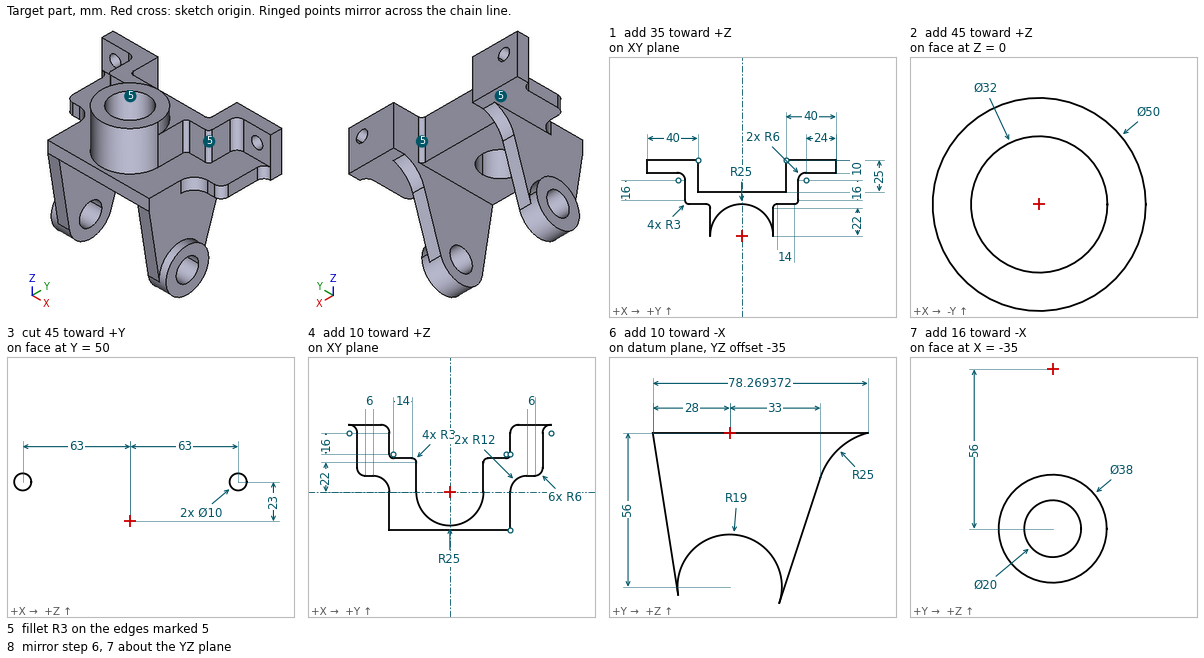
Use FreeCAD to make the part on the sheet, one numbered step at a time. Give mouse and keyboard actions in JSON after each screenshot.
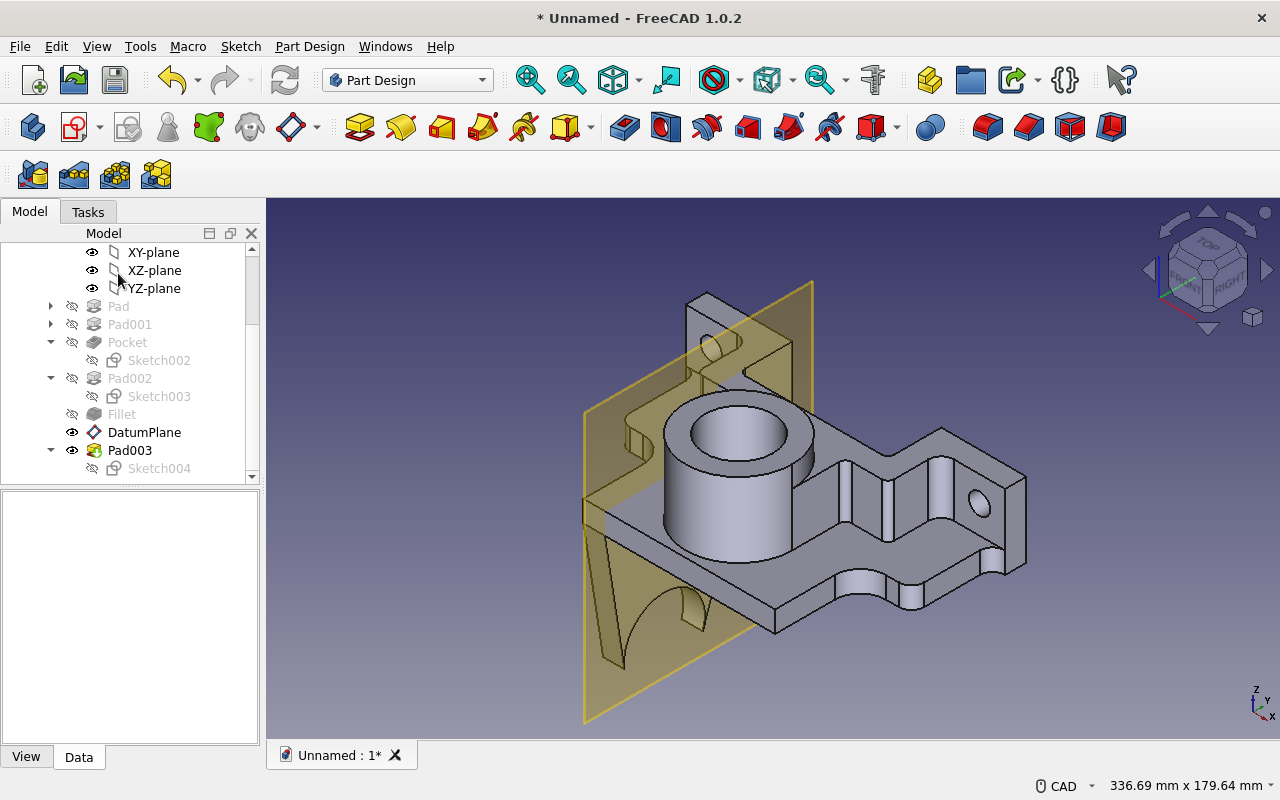
{"action": "left_click", "coordinate": [117, 432]}
{"action": "key", "text": "space"}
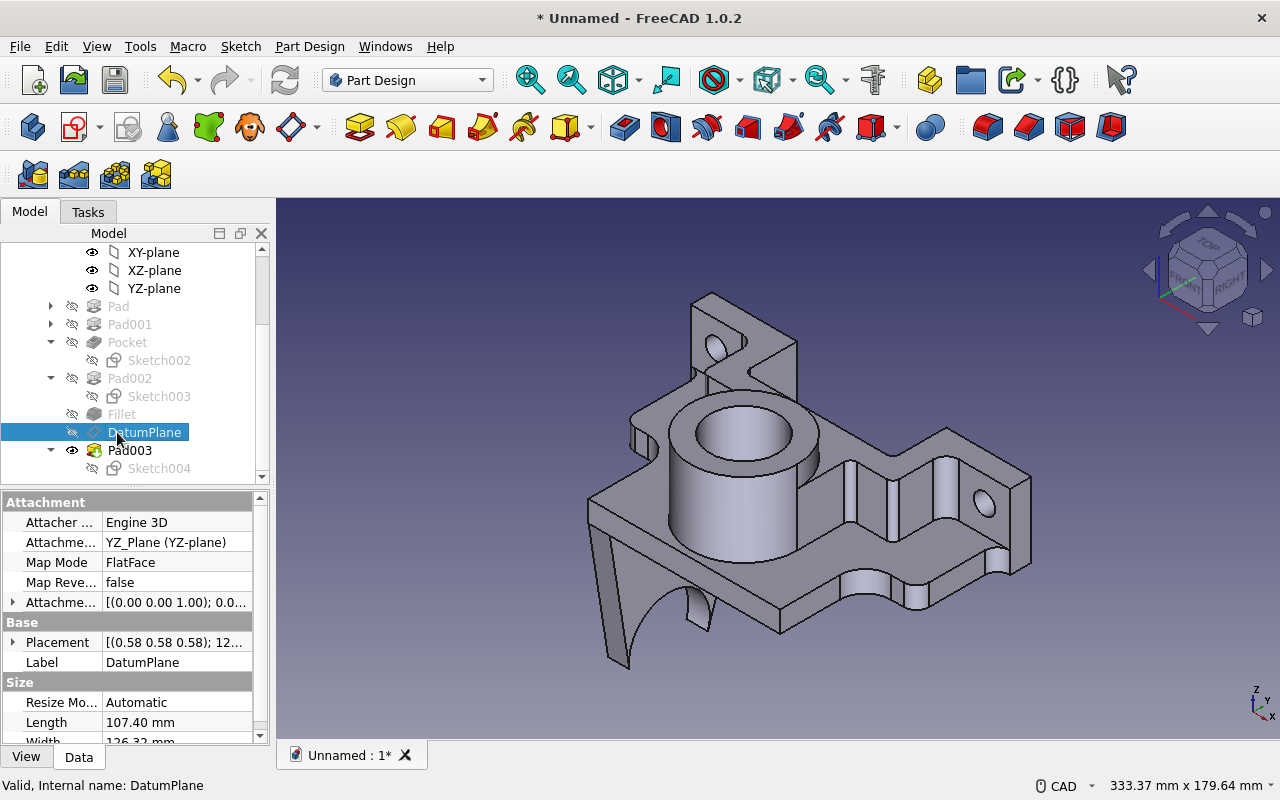
{"action": "left_click", "coordinate": [531, 80]}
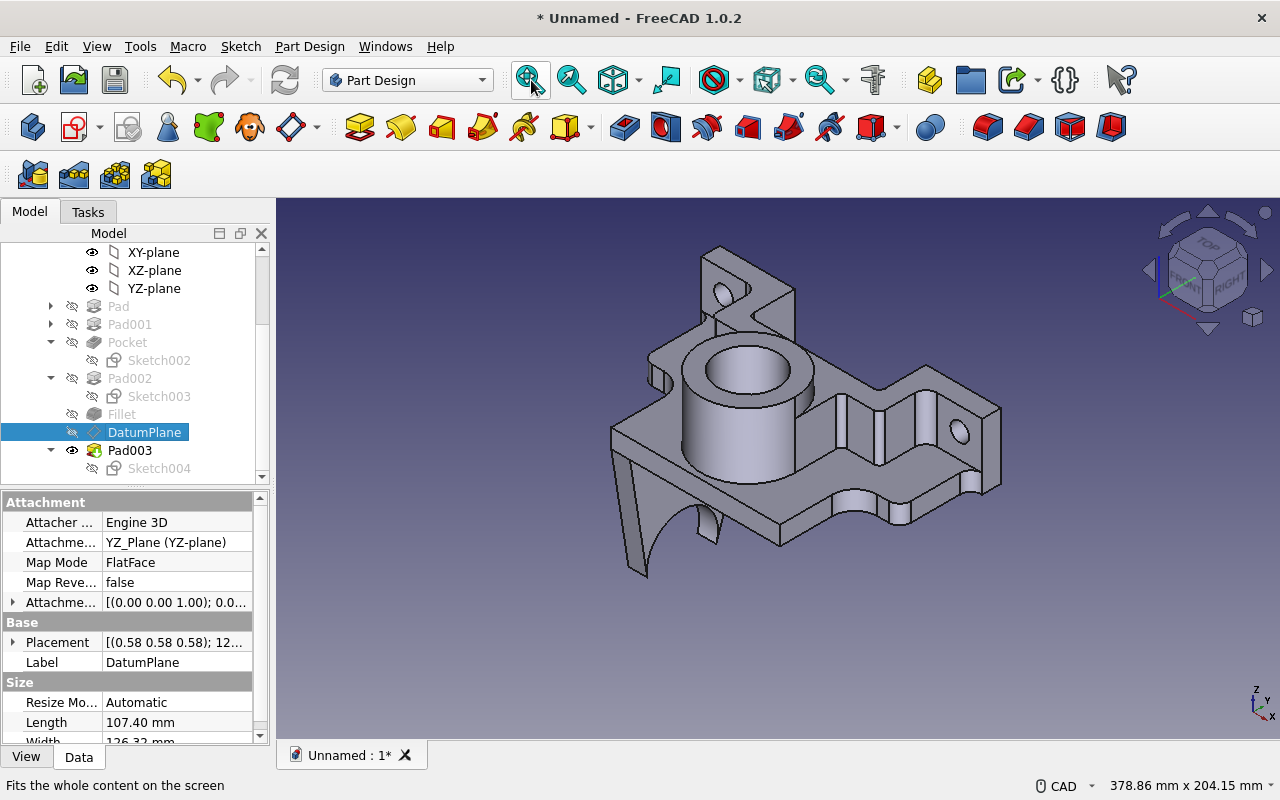
{"action": "left_click", "coordinate": [665, 498]}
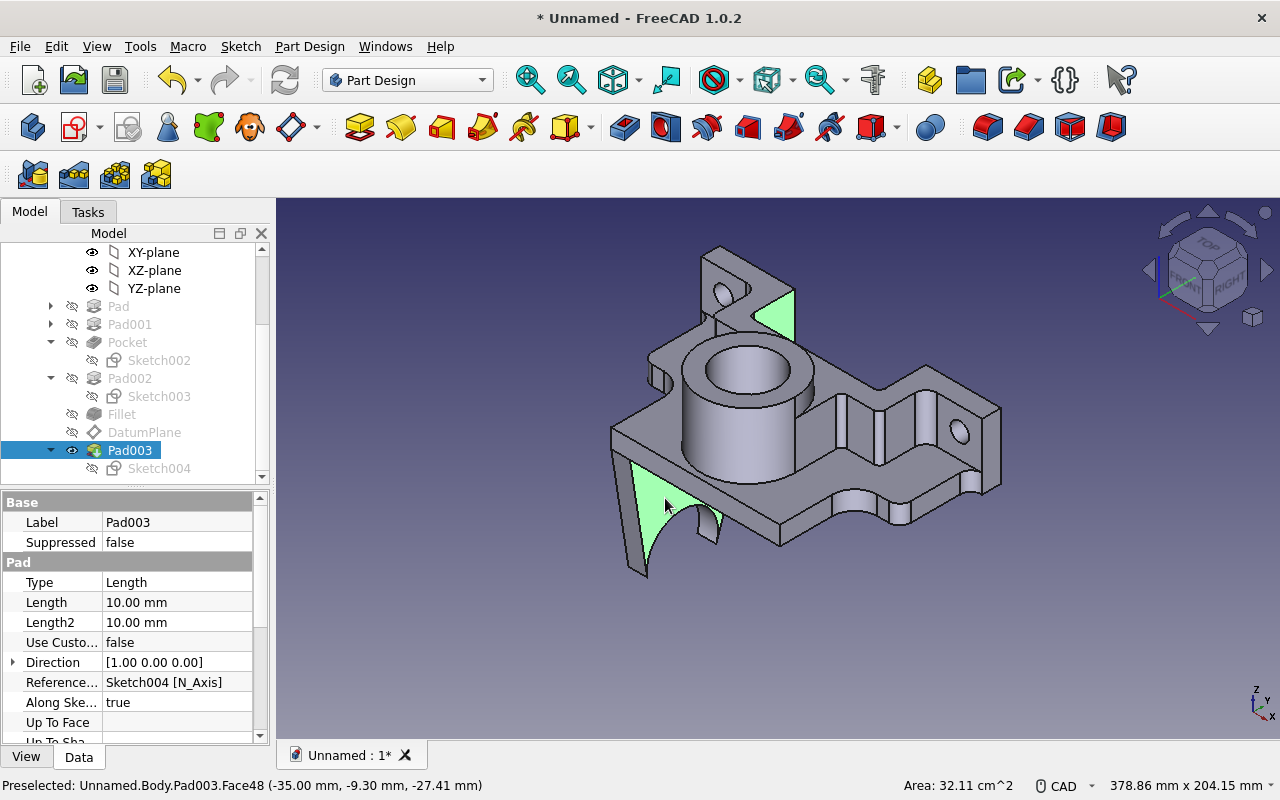
{"action": "left_click", "coordinate": [74, 128]}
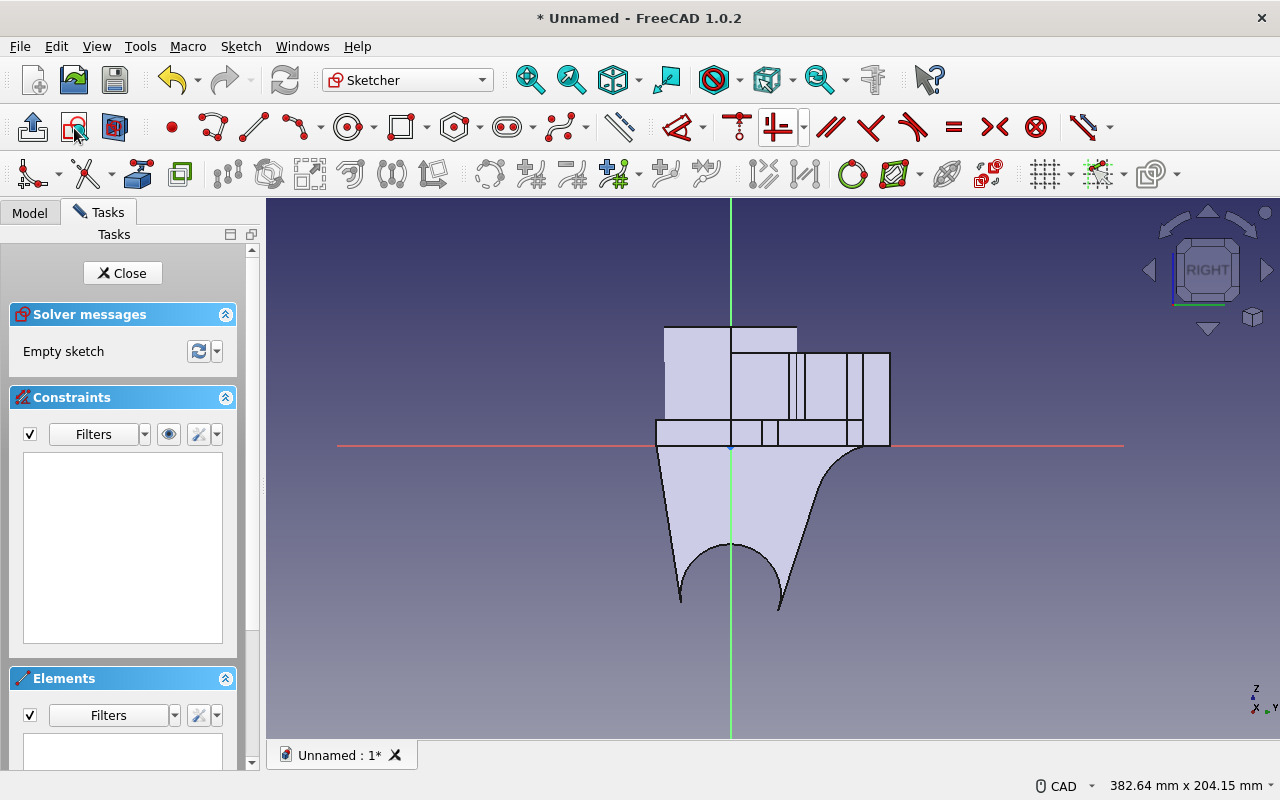
{"action": "scroll", "coordinate": [762, 639], "scroll_direction": "up", "scroll_amount": 3}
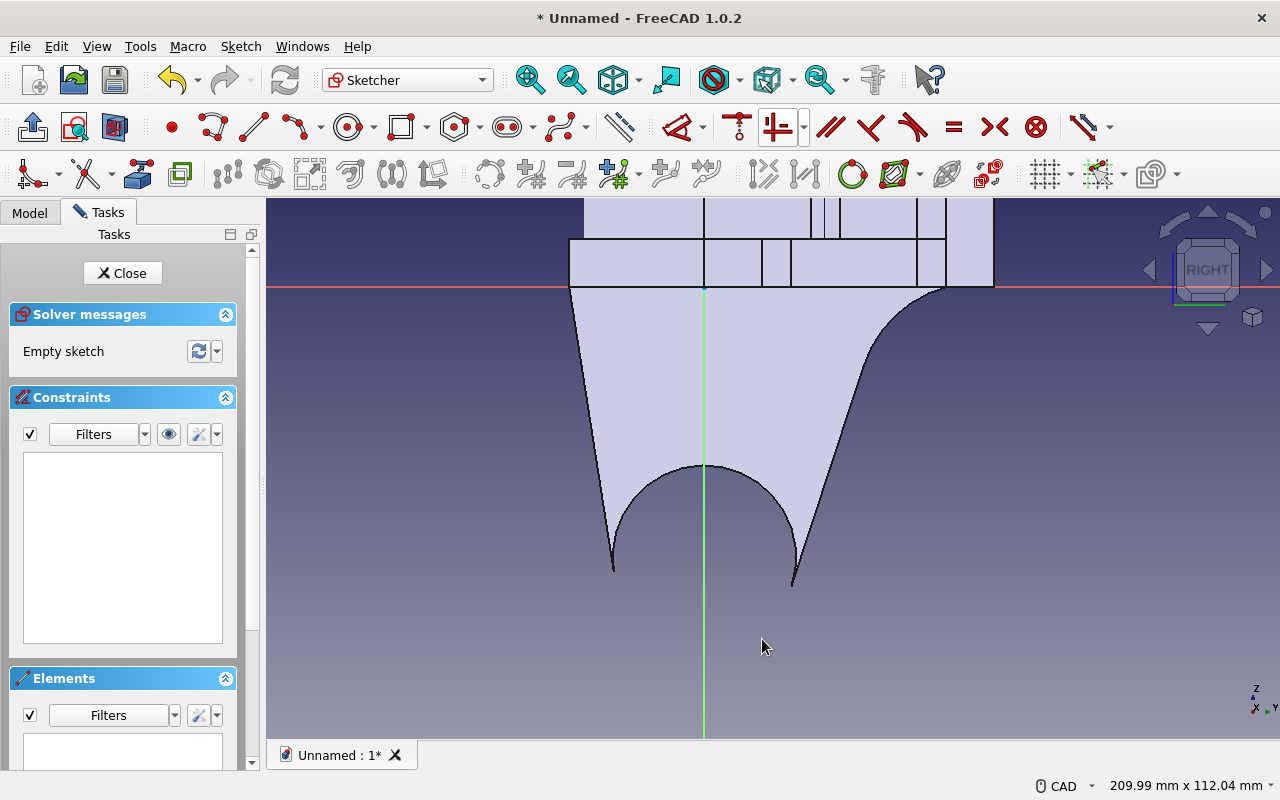
{"action": "left_click", "coordinate": [348, 128]}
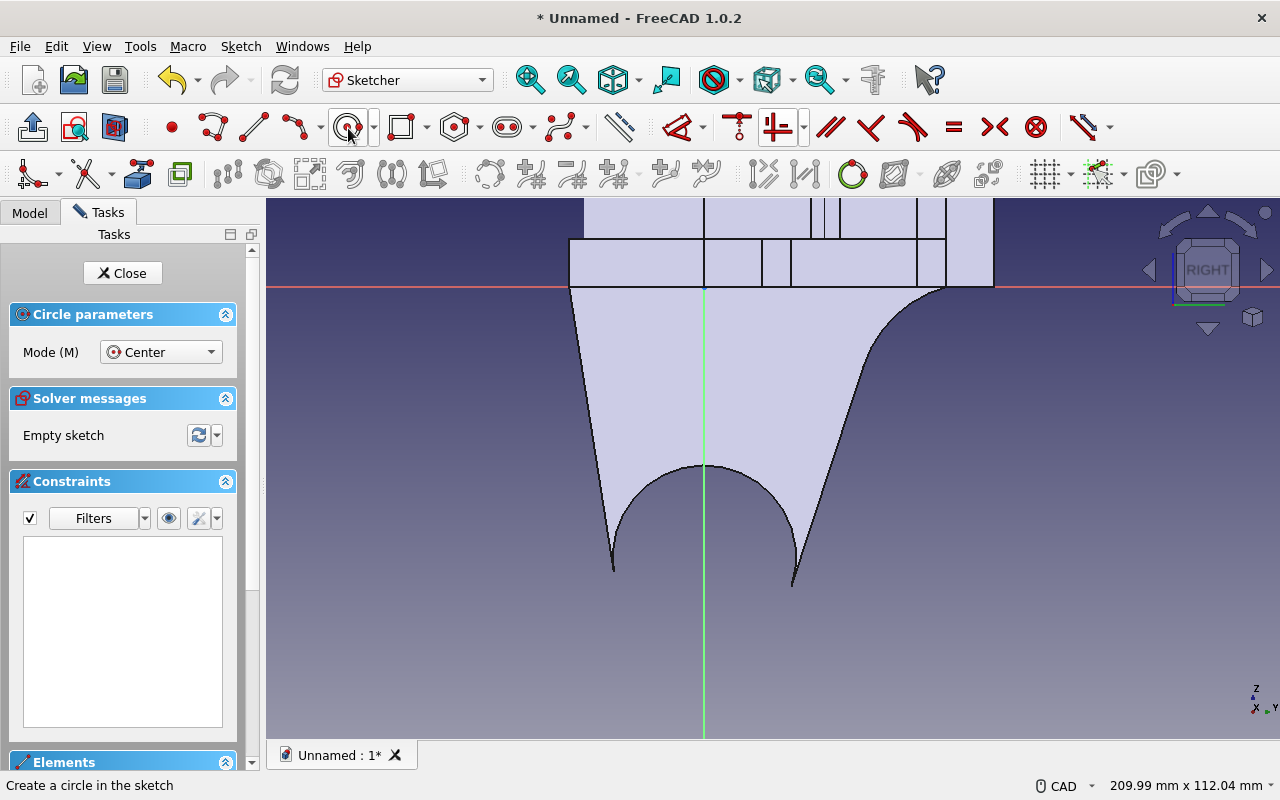
{"action": "left_click", "coordinate": [704, 557]}
{"action": "left_click", "coordinate": [769, 492]}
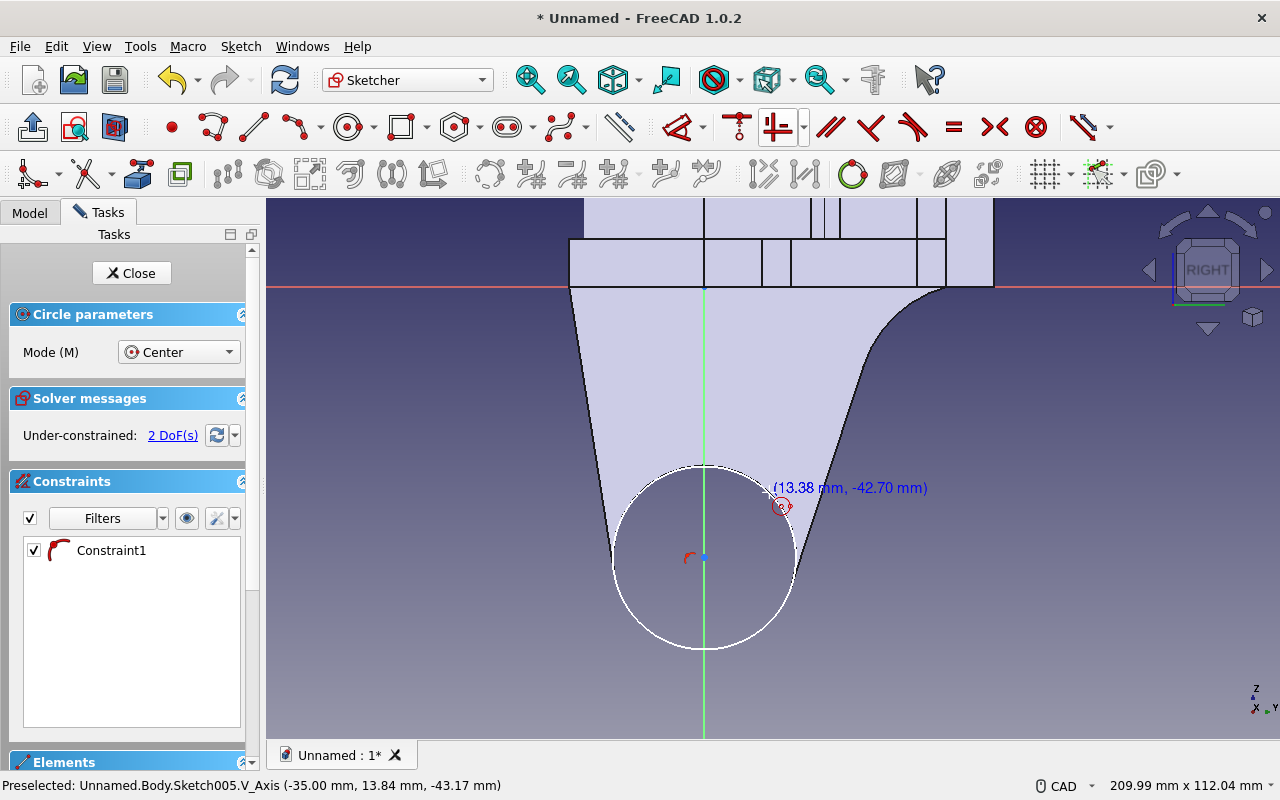
{"action": "left_click", "coordinate": [704, 558]}
{"action": "left_click", "coordinate": [739, 523]}
{"action": "key", "text": "Escape"}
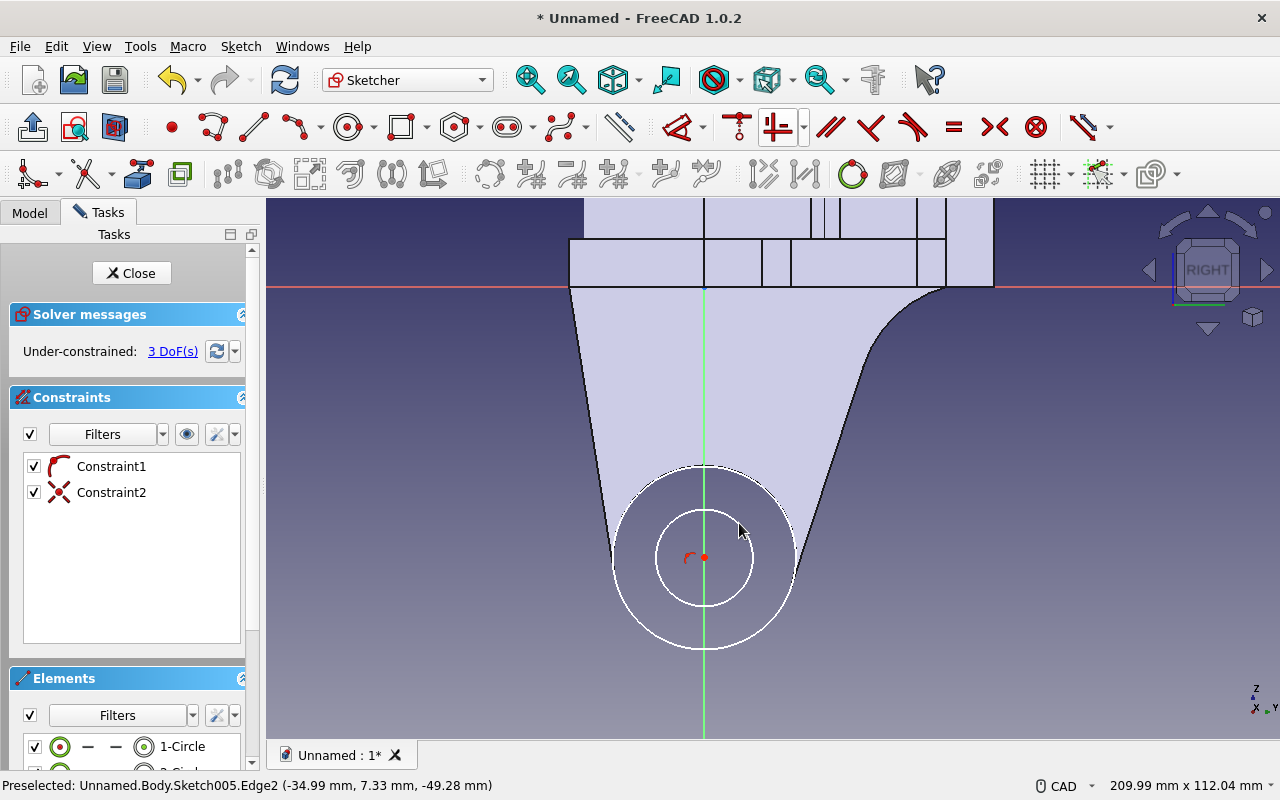
{"action": "left_click", "coordinate": [676, 128]}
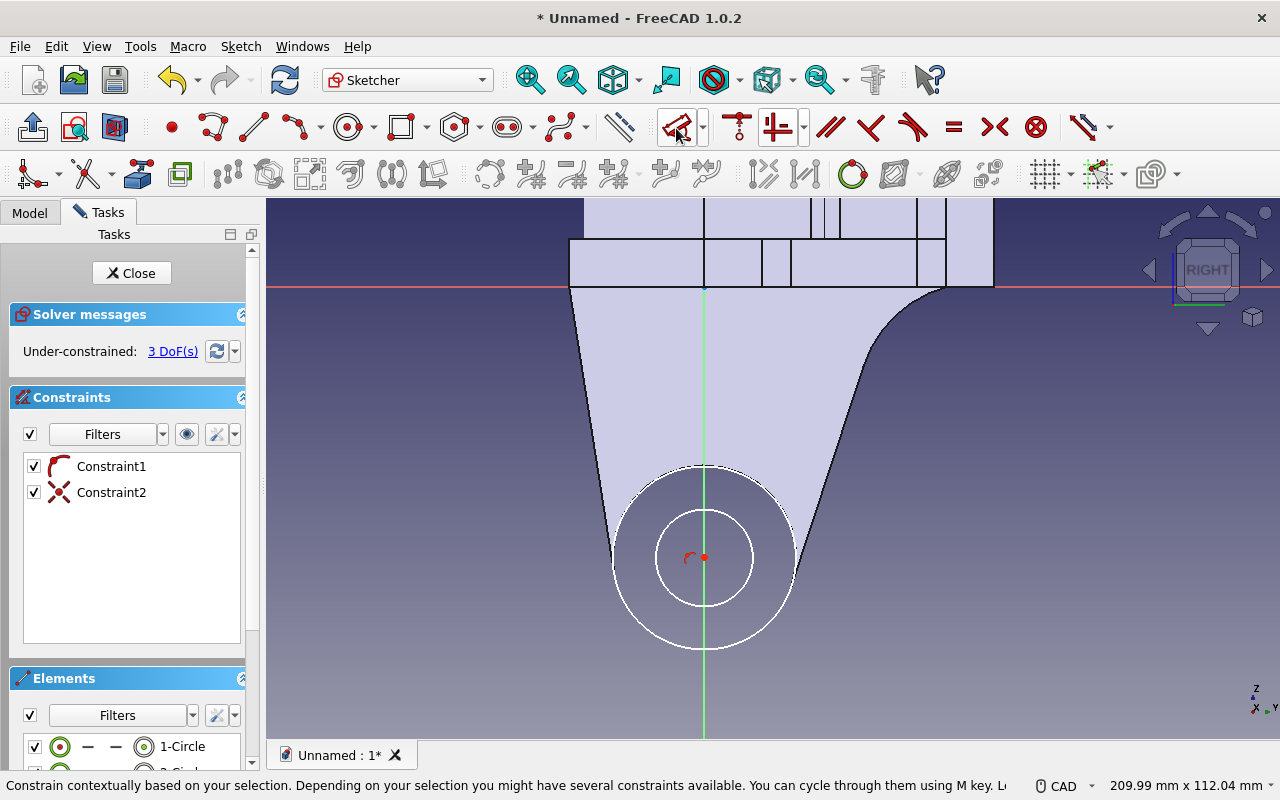
{"action": "left_click", "coordinate": [769, 493]}
{"action": "left_click", "coordinate": [792, 470]}